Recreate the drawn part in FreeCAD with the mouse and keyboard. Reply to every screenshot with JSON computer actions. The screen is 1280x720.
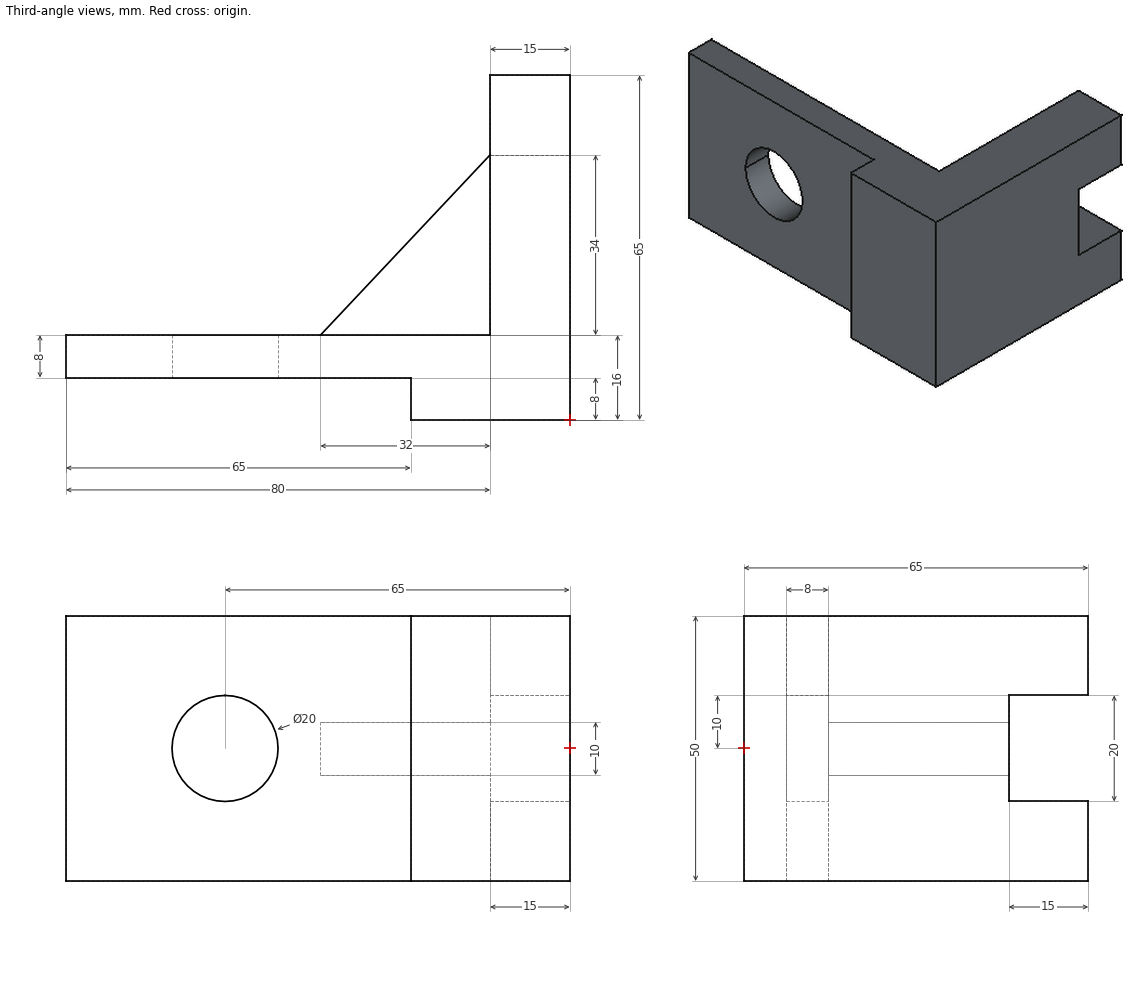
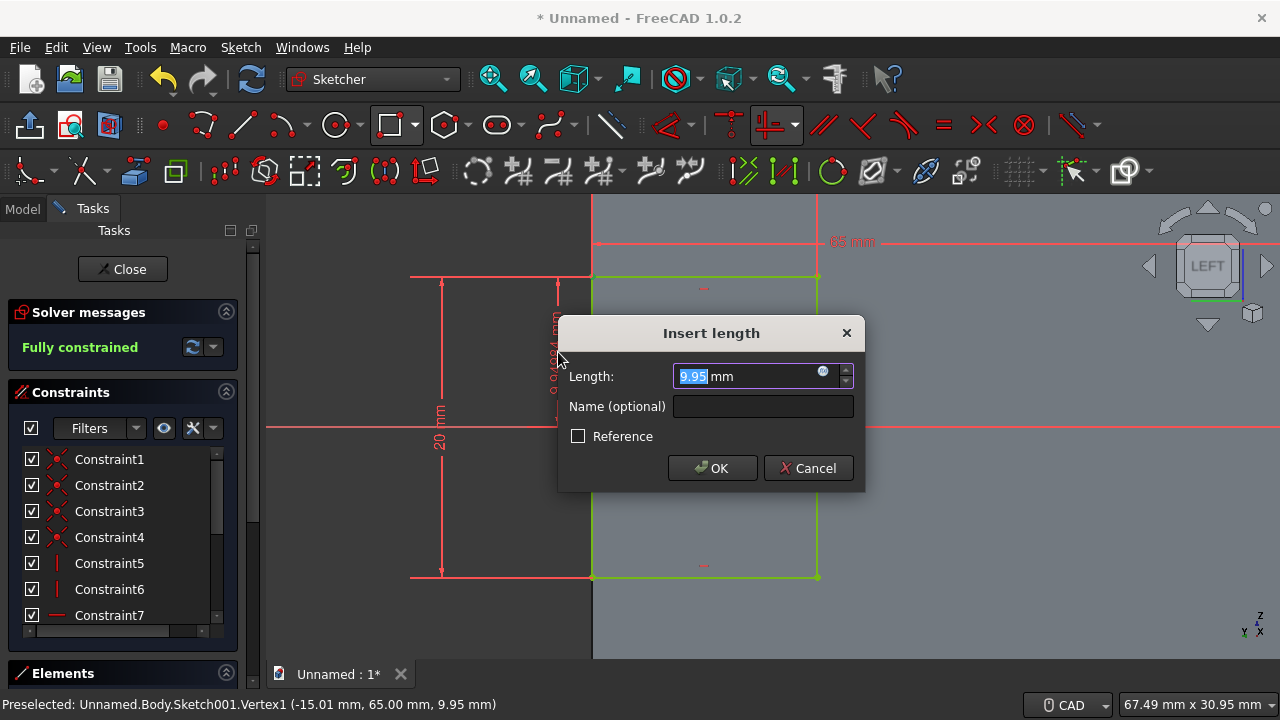
{"action": "type", "text": "10"}
{"action": "key", "text": "Return"}
{"action": "key", "text": "Escape"}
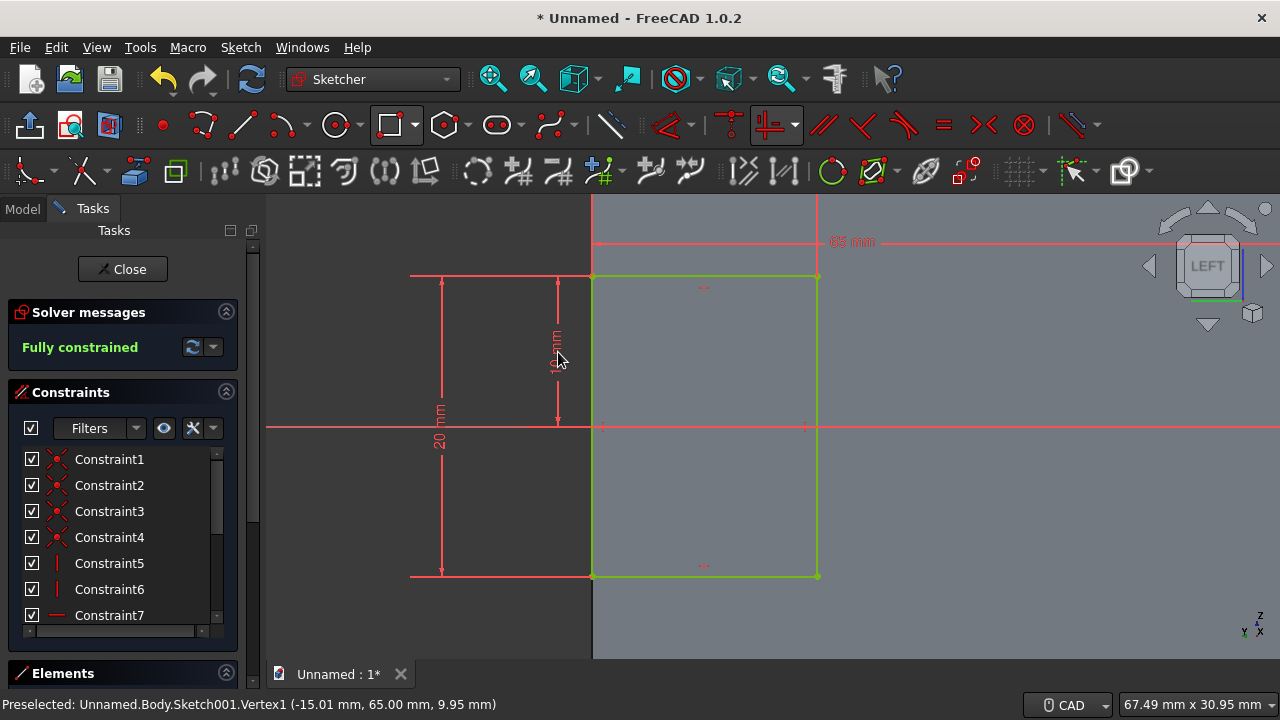
{"action": "left_click", "coordinate": [123, 269]}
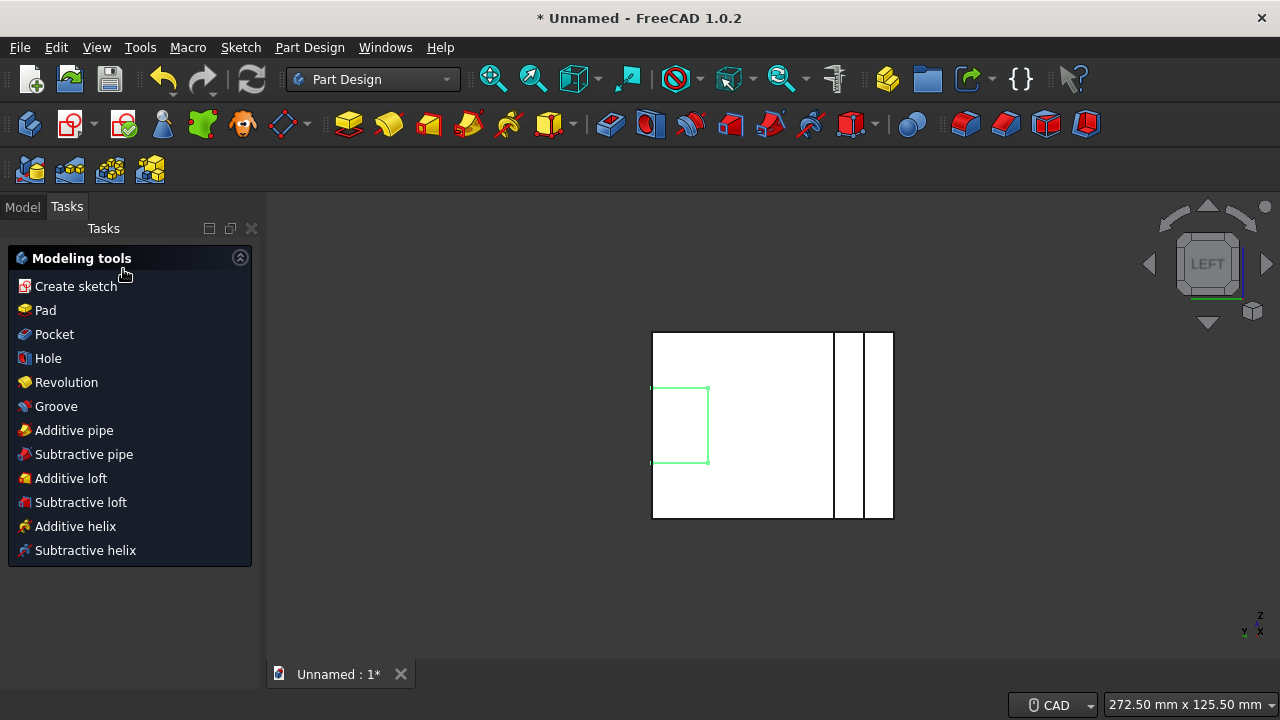
{"action": "left_click", "coordinate": [612, 124]}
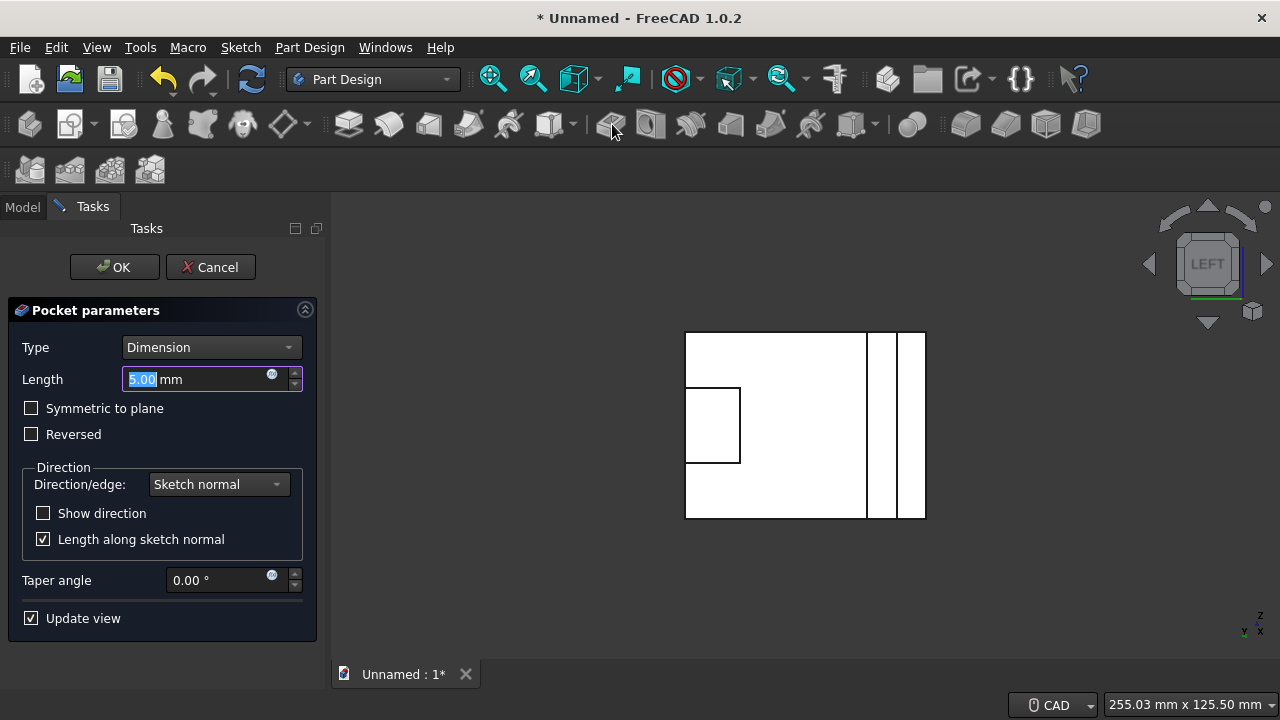
{"action": "type", "text": "15"}
{"action": "key", "text": "Tab"}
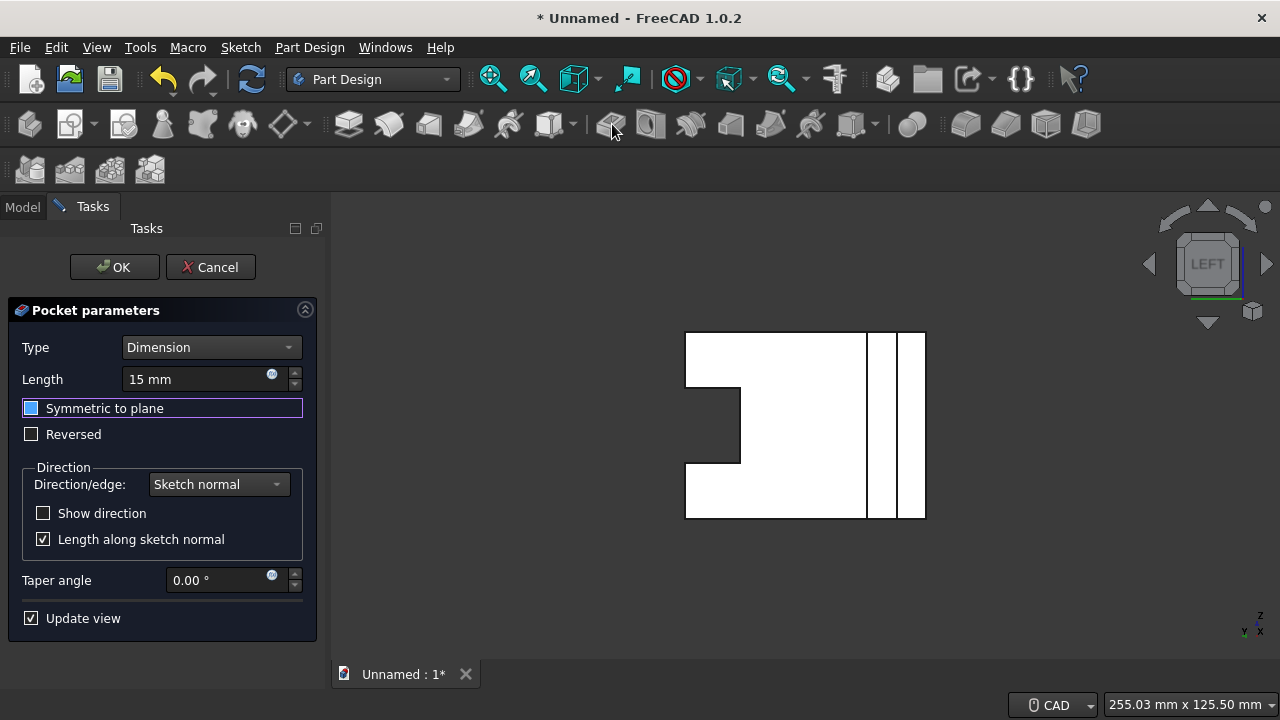
{"action": "left_click", "coordinate": [115, 267]}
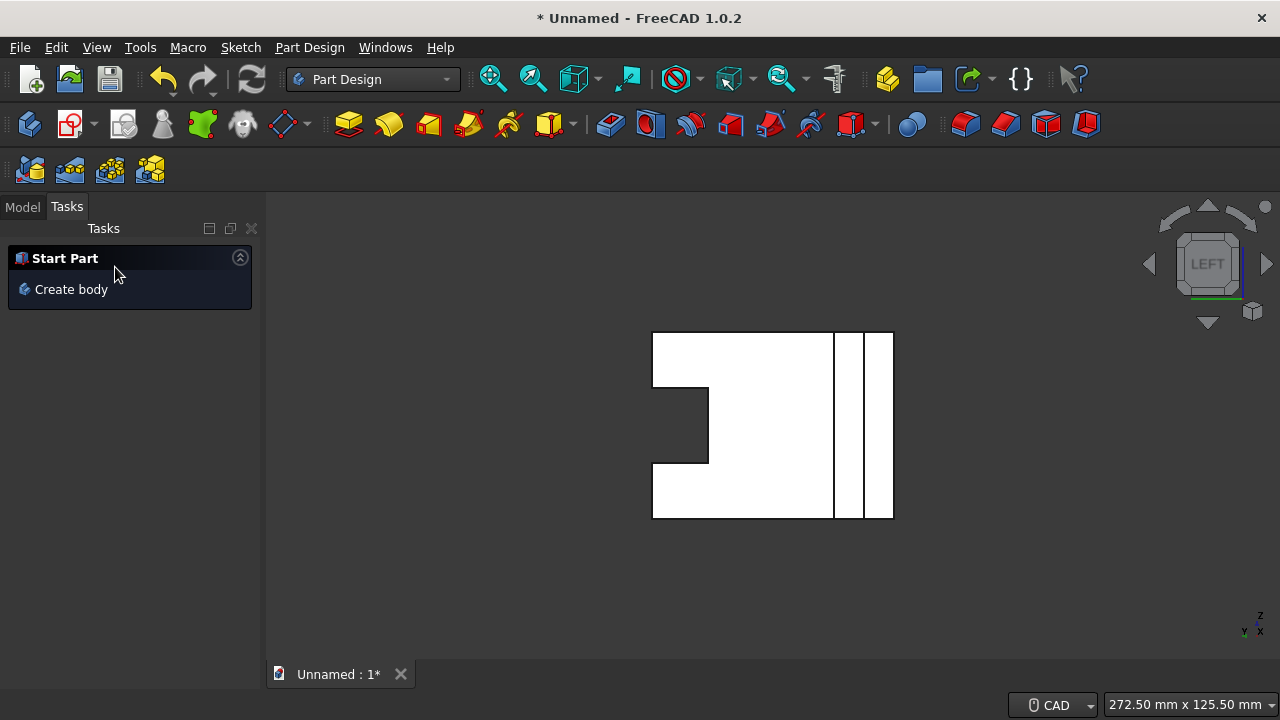
{"action": "key", "text": "v f"}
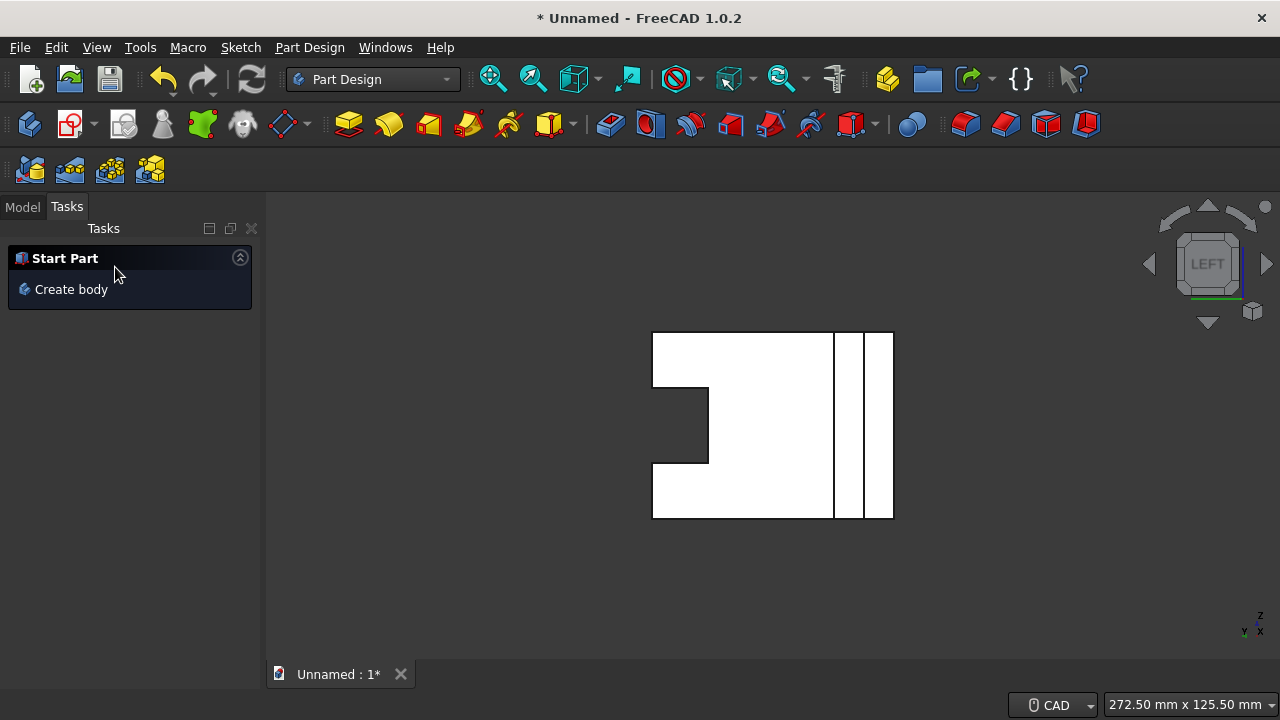
{"action": "key", "text": "4"}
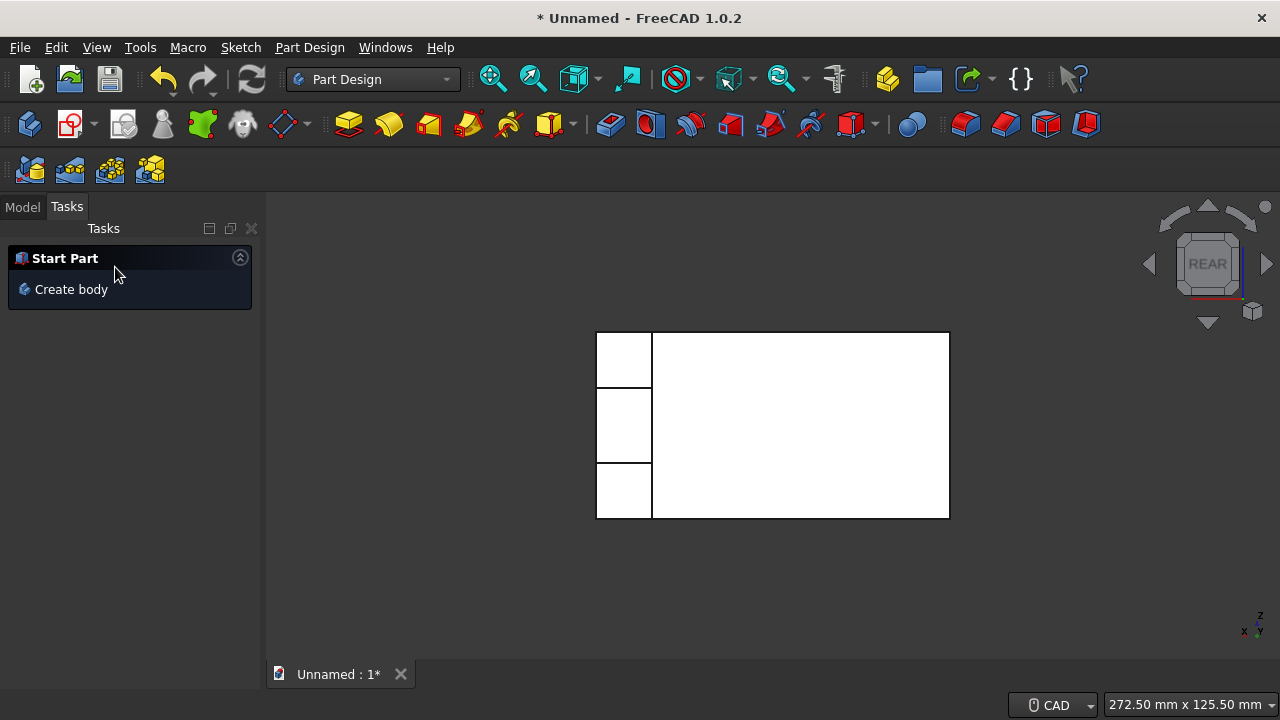
{"action": "left_click", "coordinate": [494, 80]}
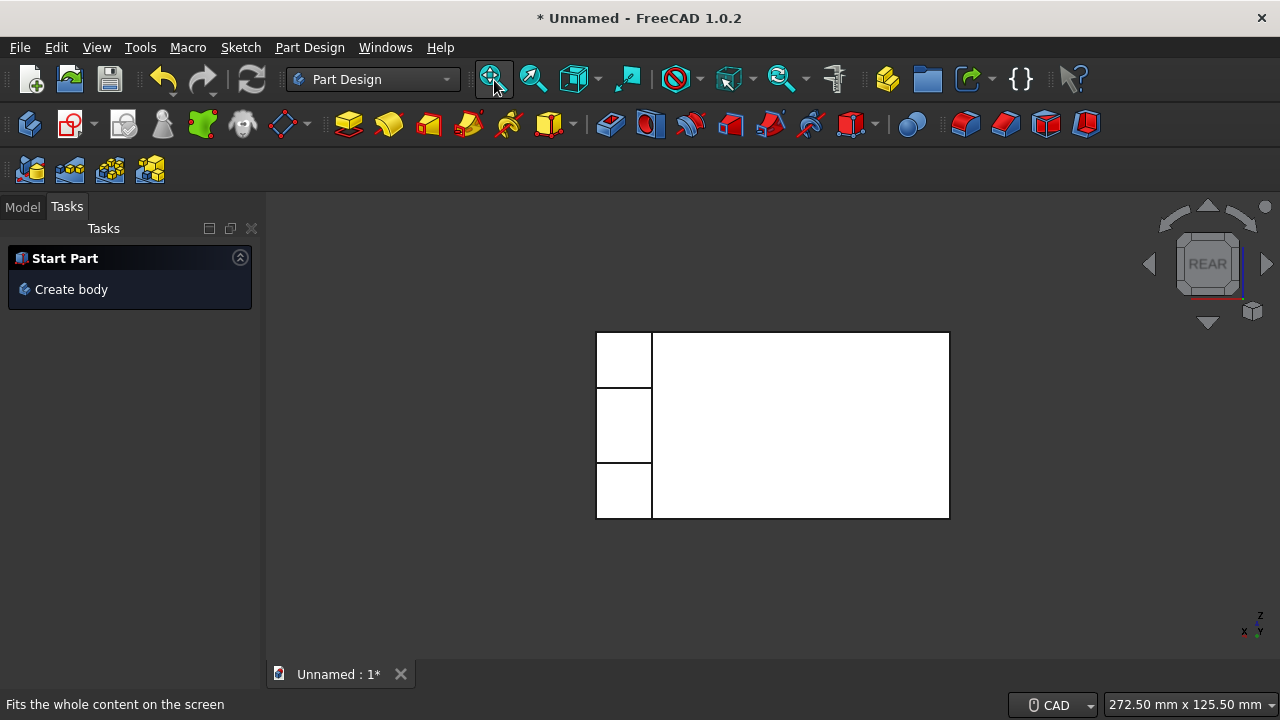
{"action": "left_click", "coordinate": [758, 425]}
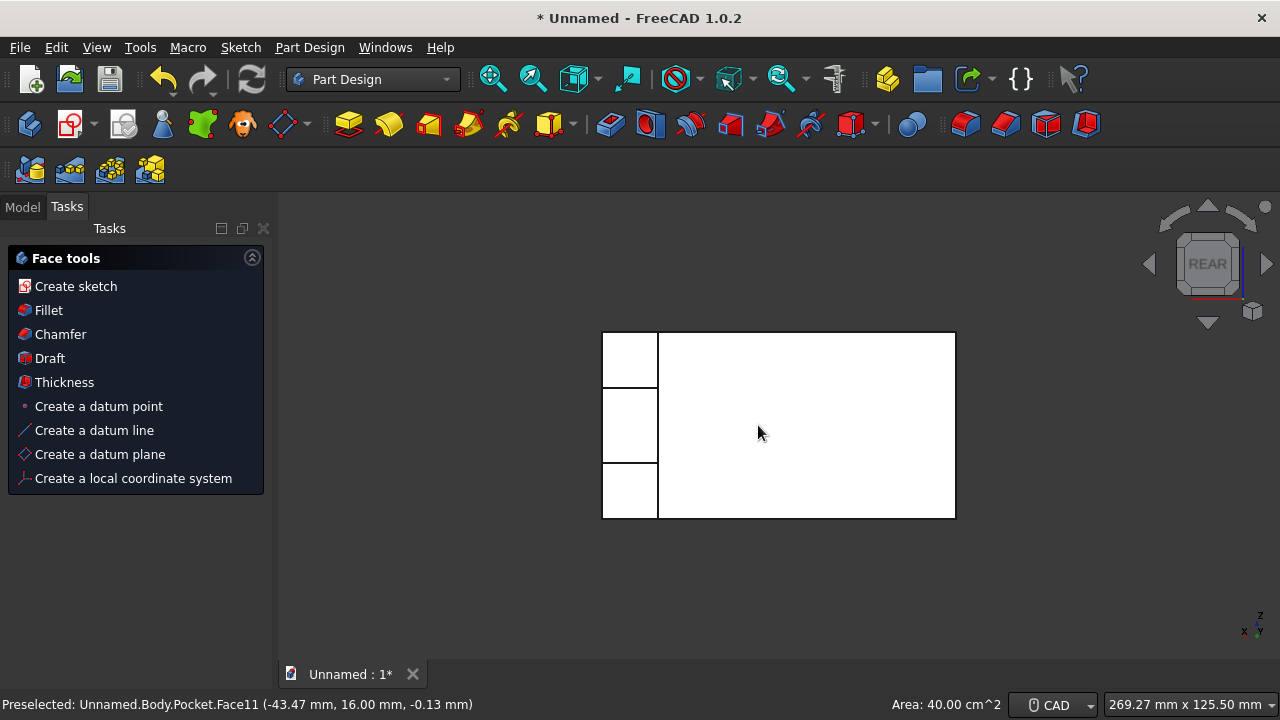
{"action": "left_click", "coordinate": [70, 124]}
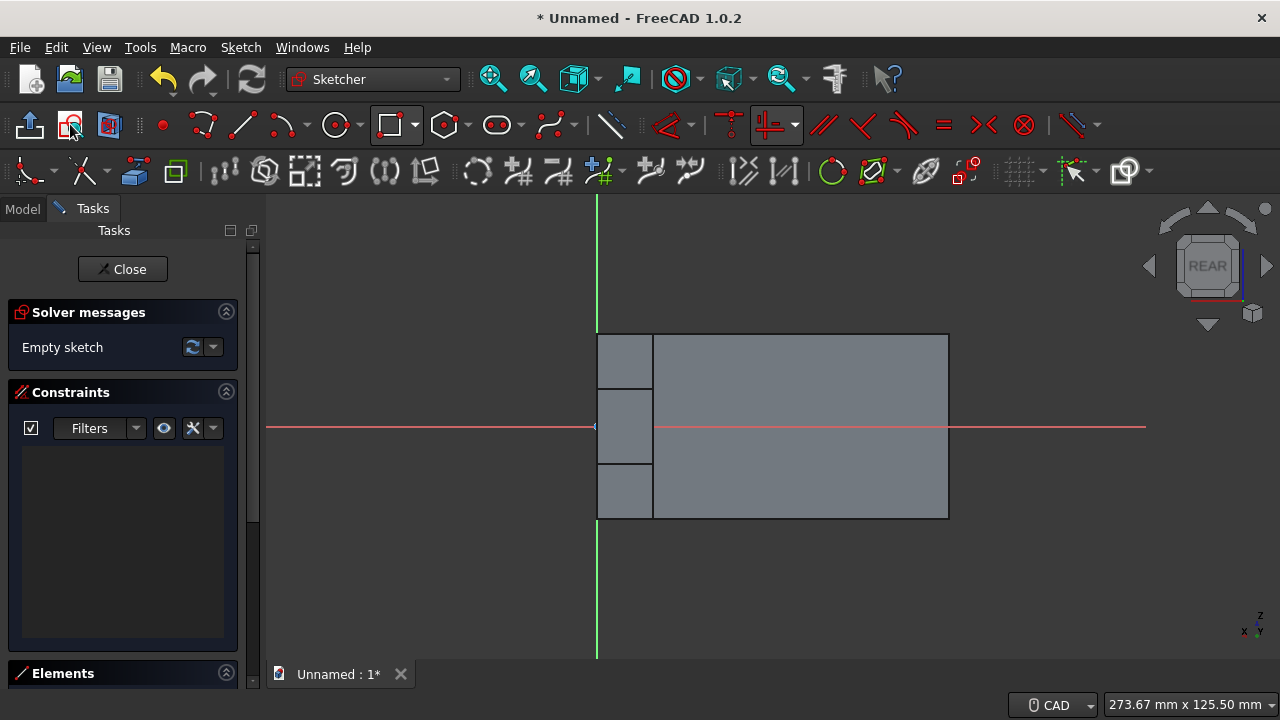
{"action": "left_click", "coordinate": [110, 126]}